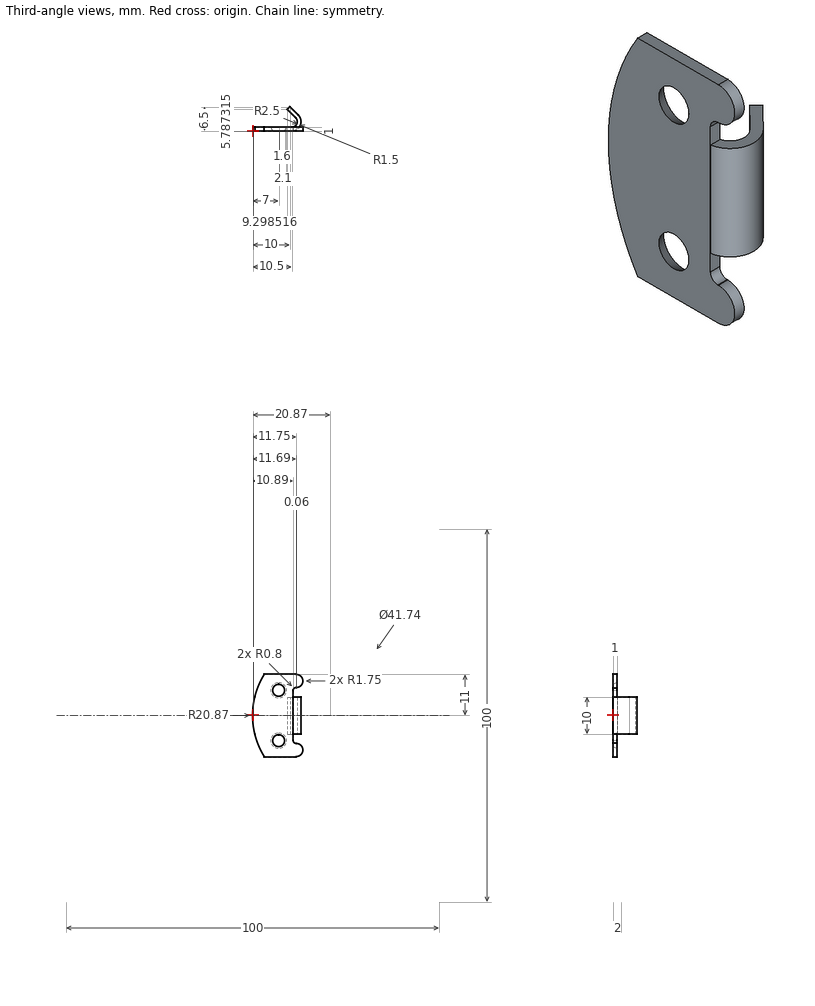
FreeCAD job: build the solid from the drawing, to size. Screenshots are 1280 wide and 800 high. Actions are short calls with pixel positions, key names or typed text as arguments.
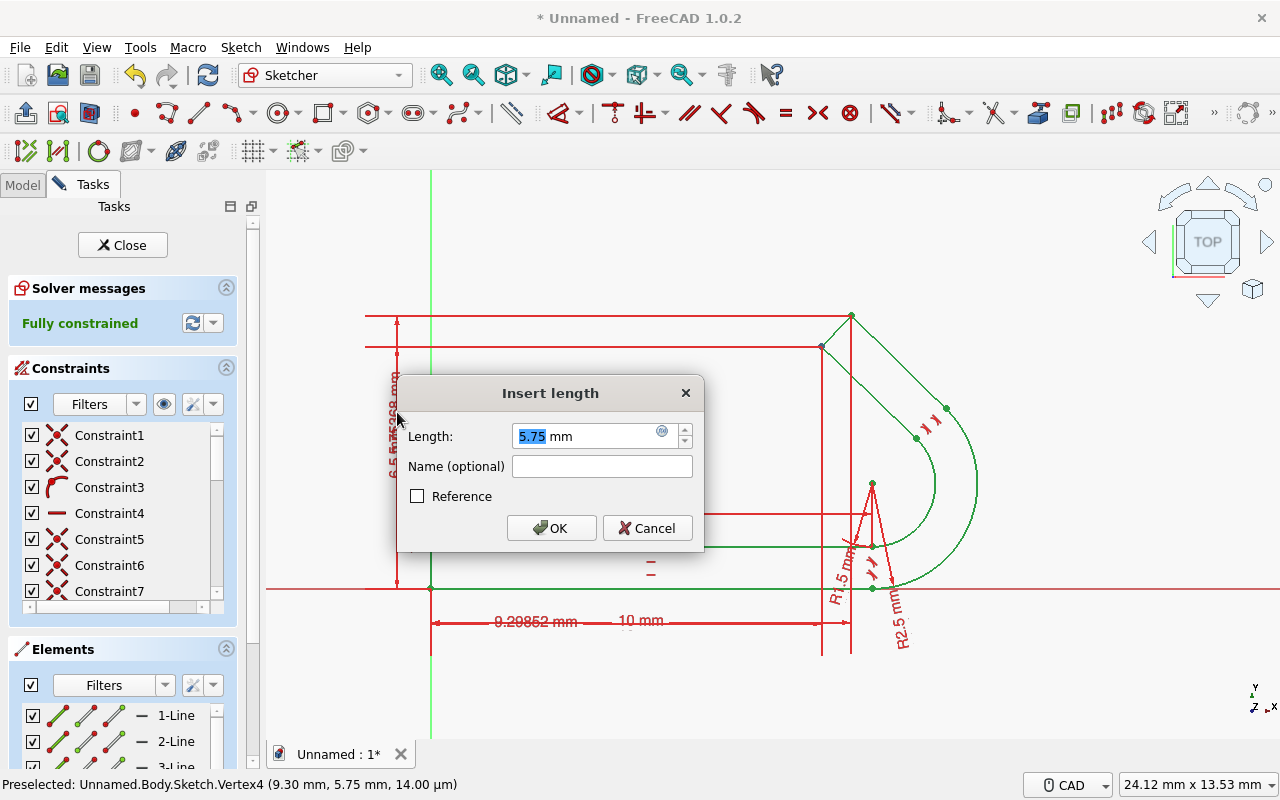
text(5.787315)
key(Return)
key(Escape)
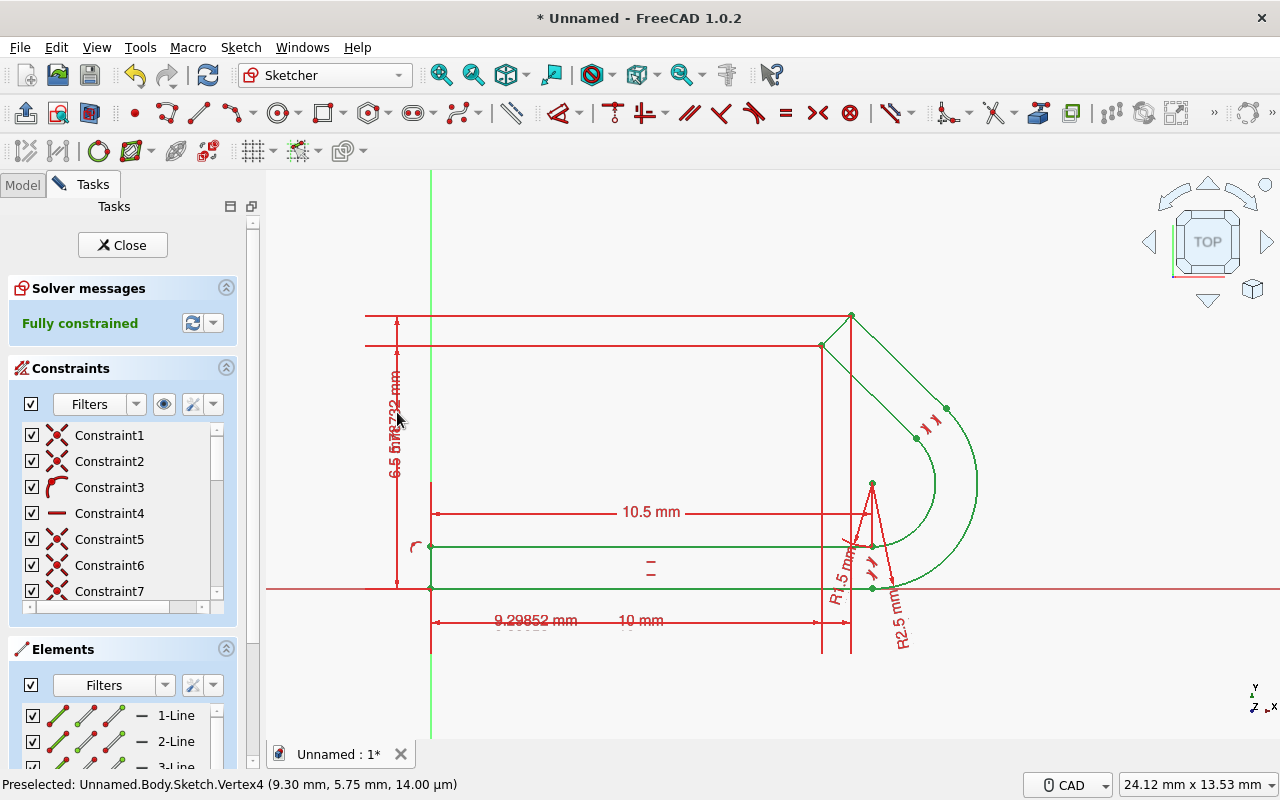
click(123, 245)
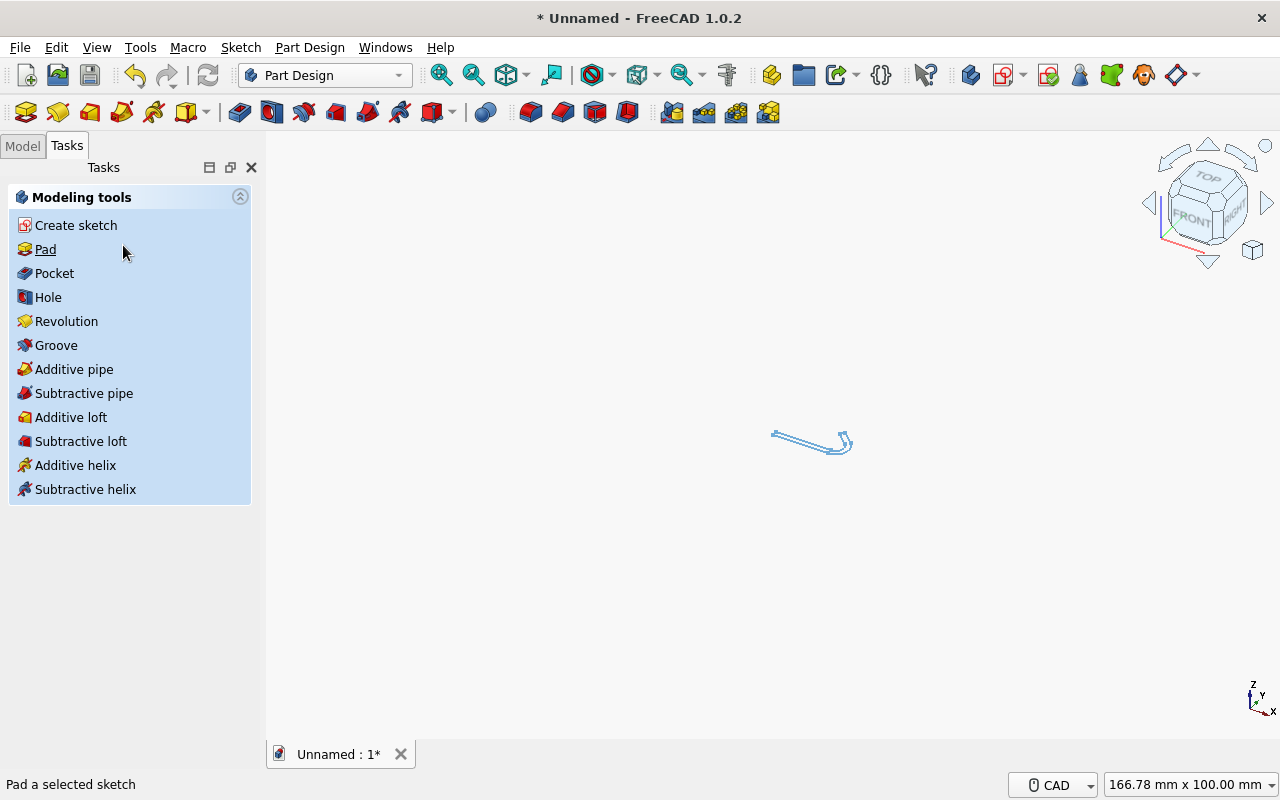
click(26, 112)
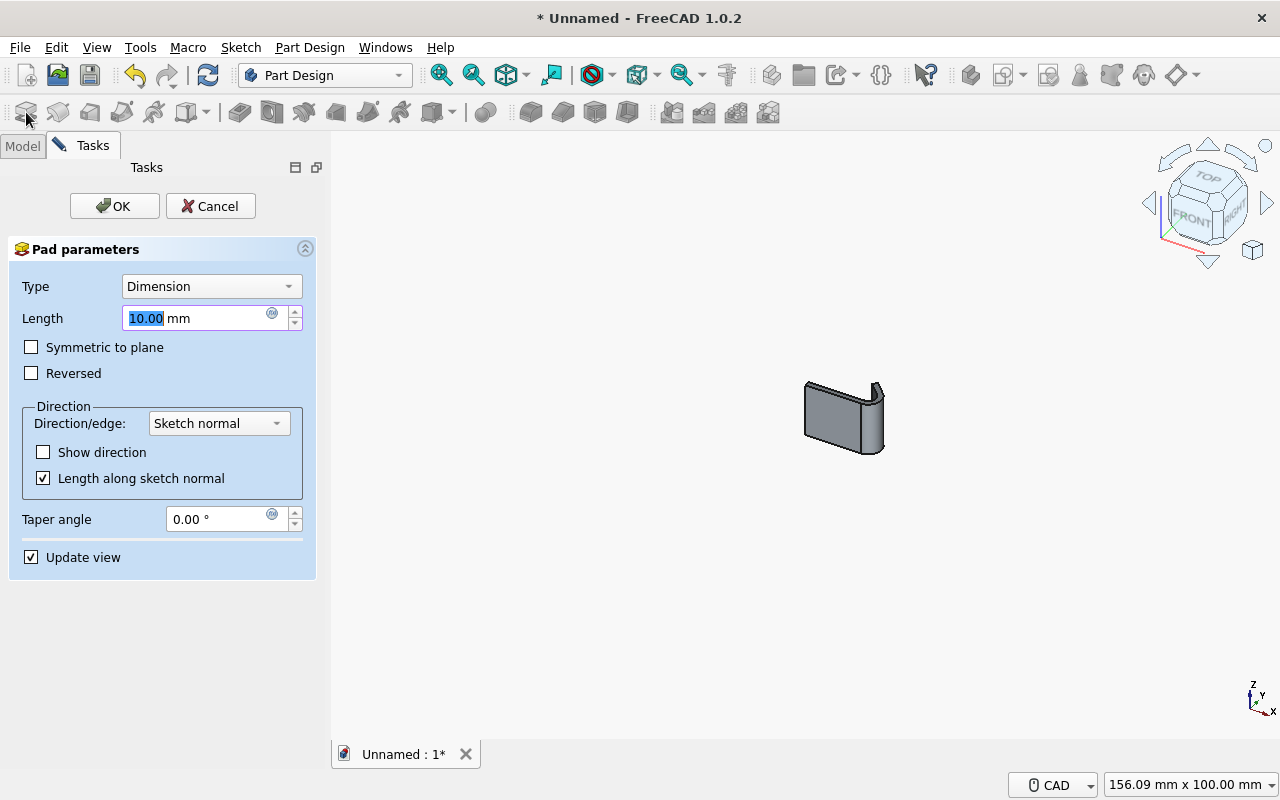
text(10)
key(Tab)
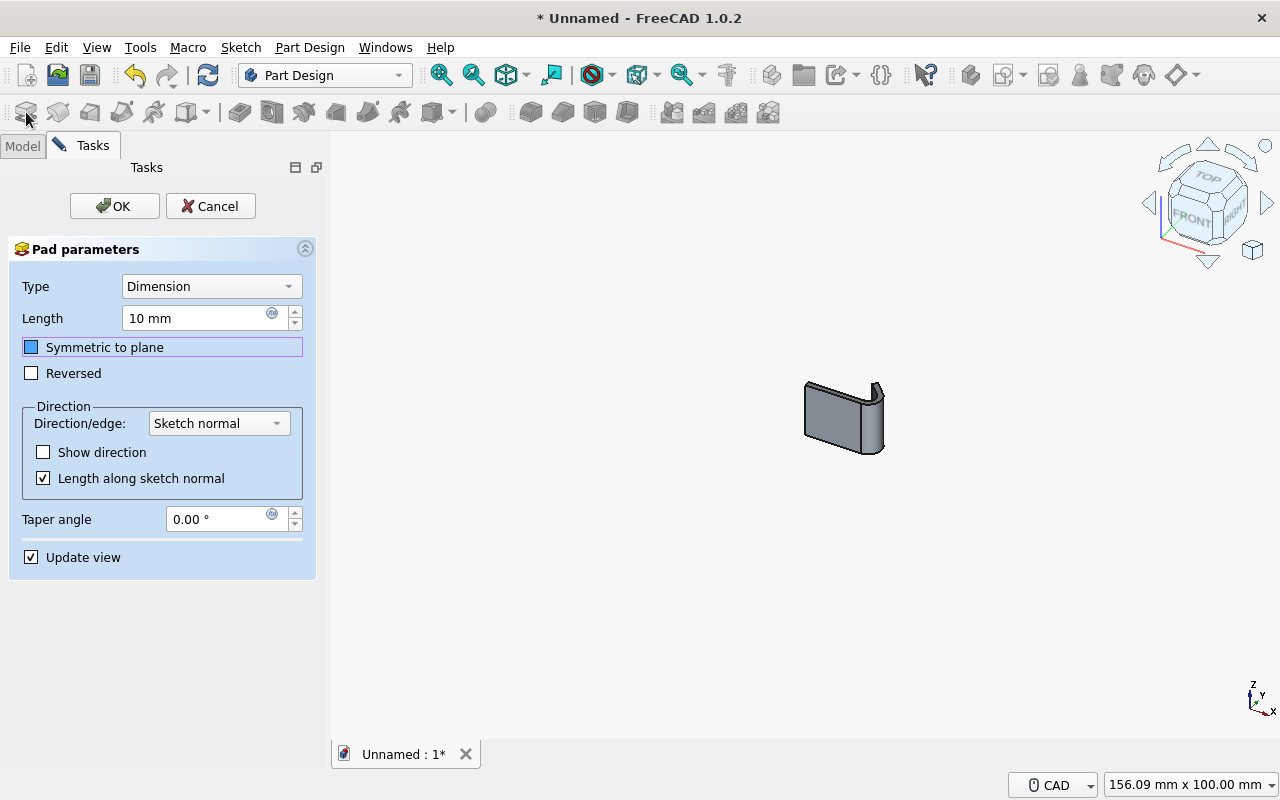
click(30, 347)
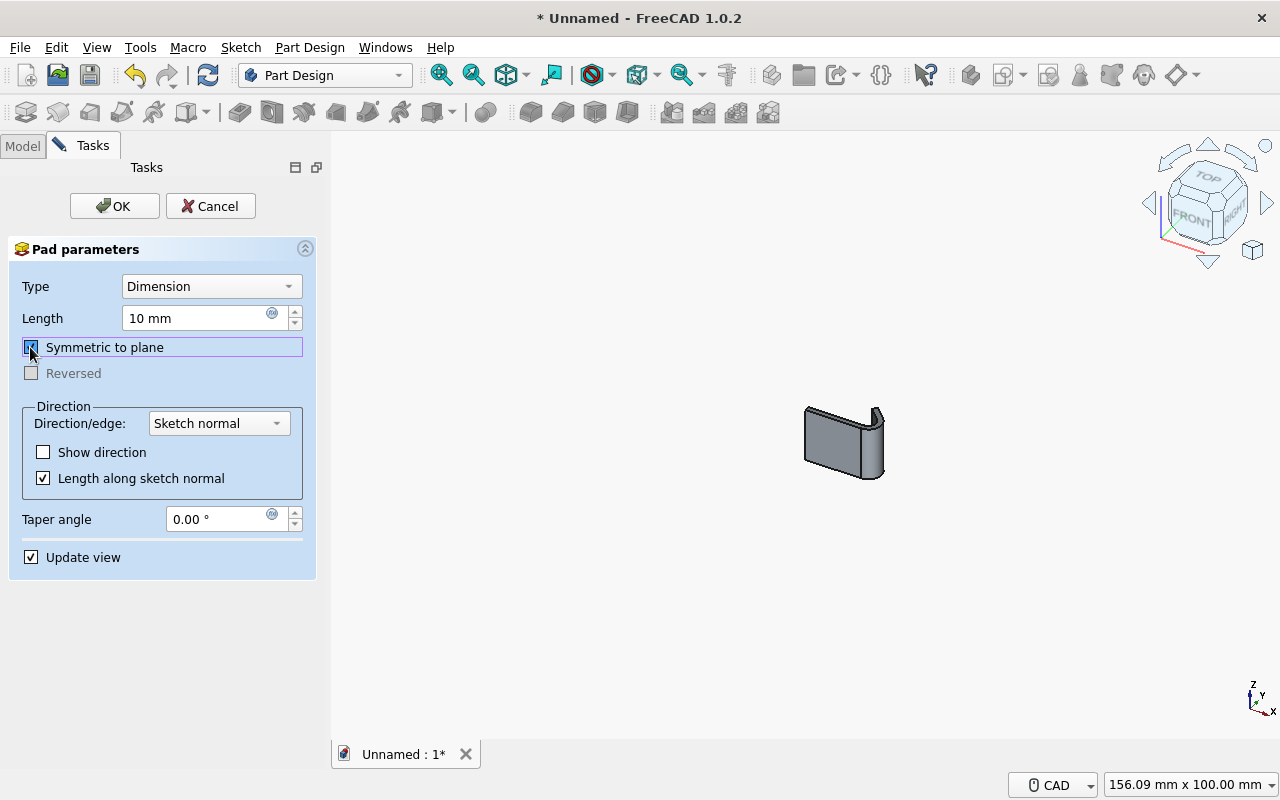
click(115, 206)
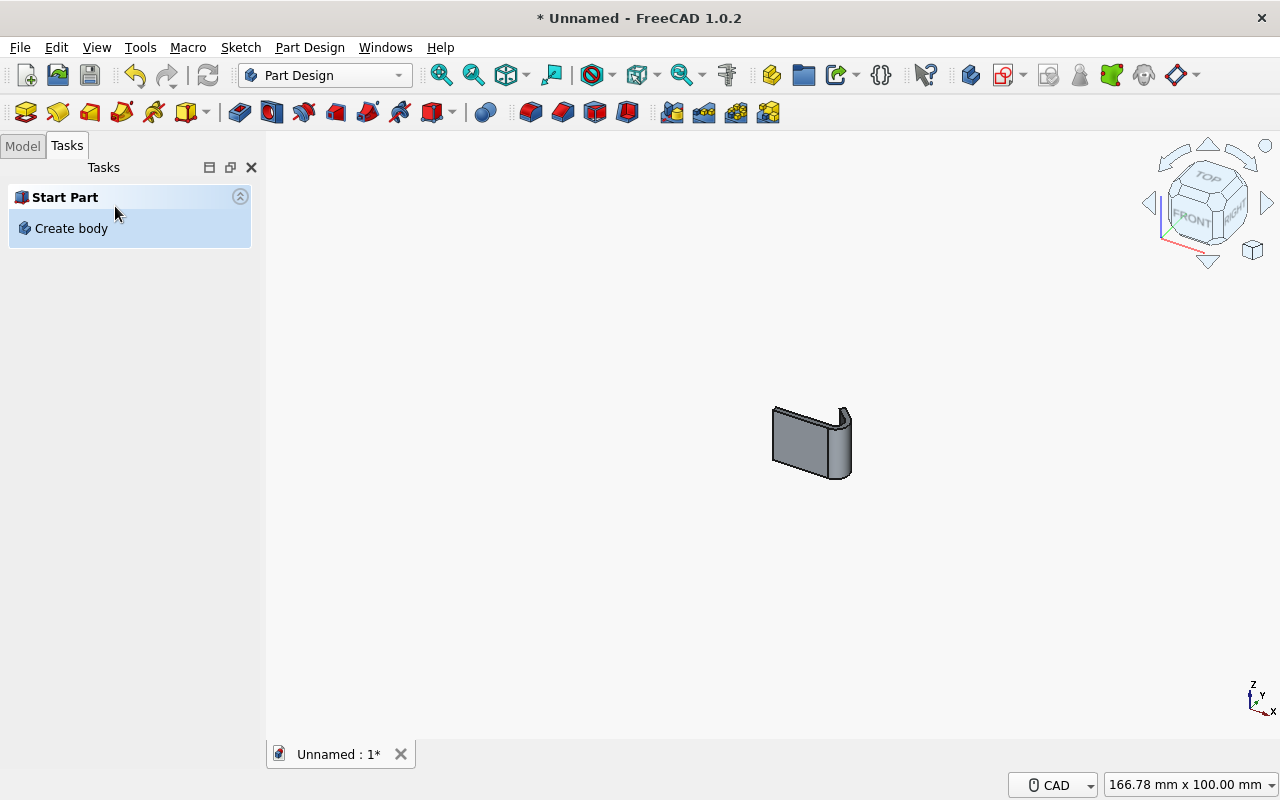
click(442, 76)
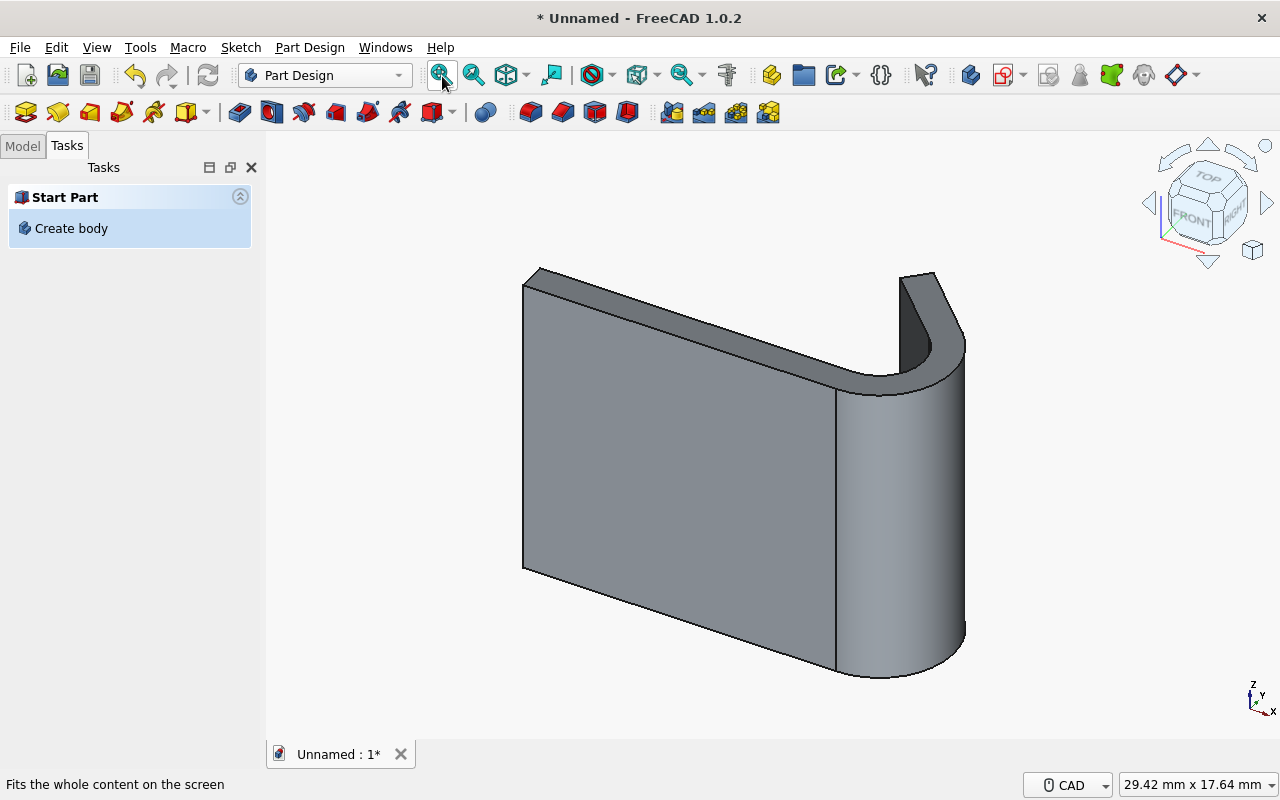
click(1004, 76)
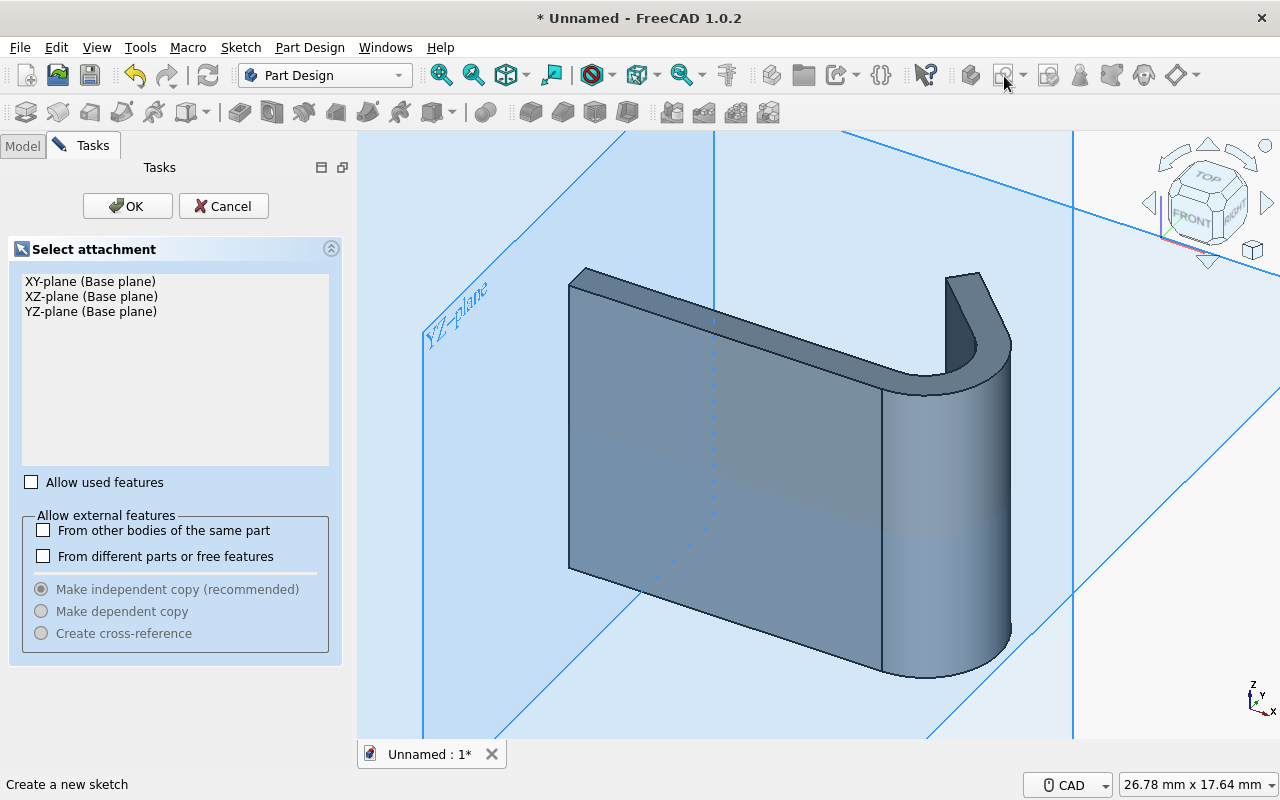
click(82, 296)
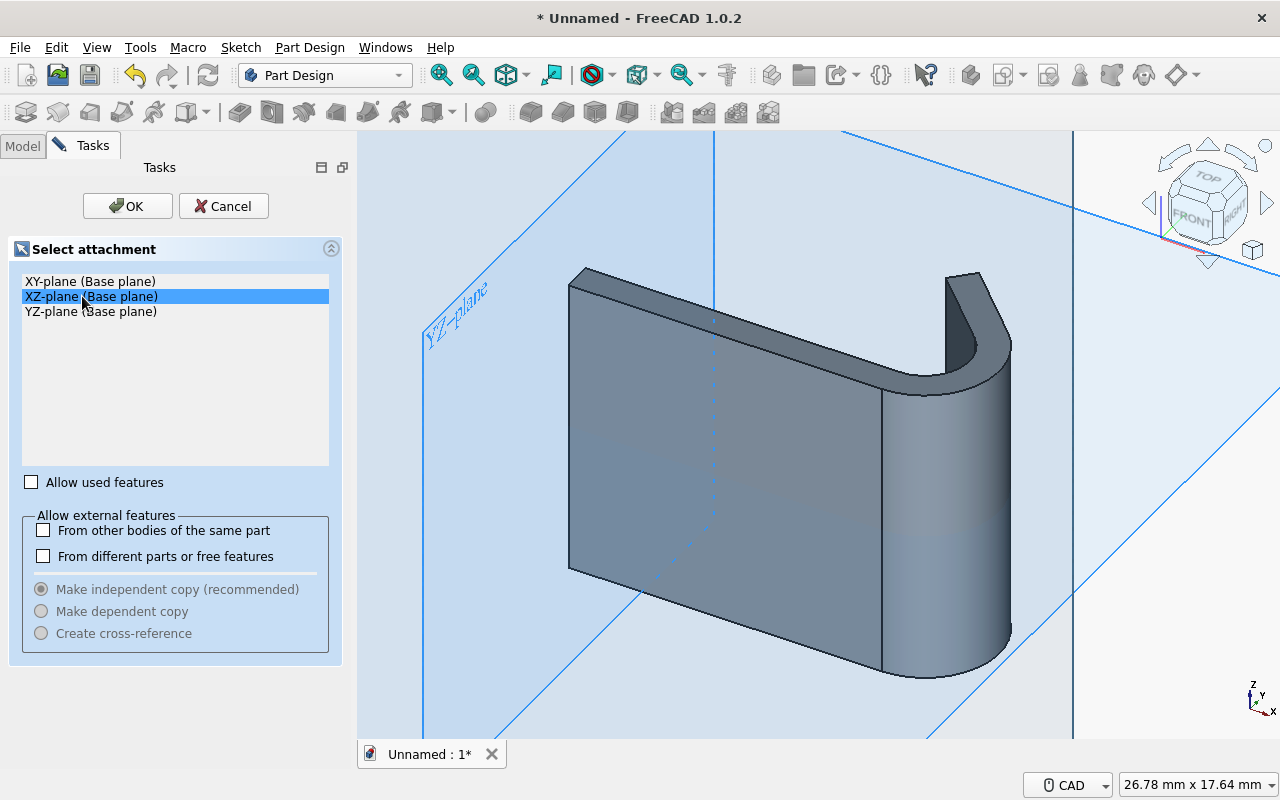
click(128, 206)